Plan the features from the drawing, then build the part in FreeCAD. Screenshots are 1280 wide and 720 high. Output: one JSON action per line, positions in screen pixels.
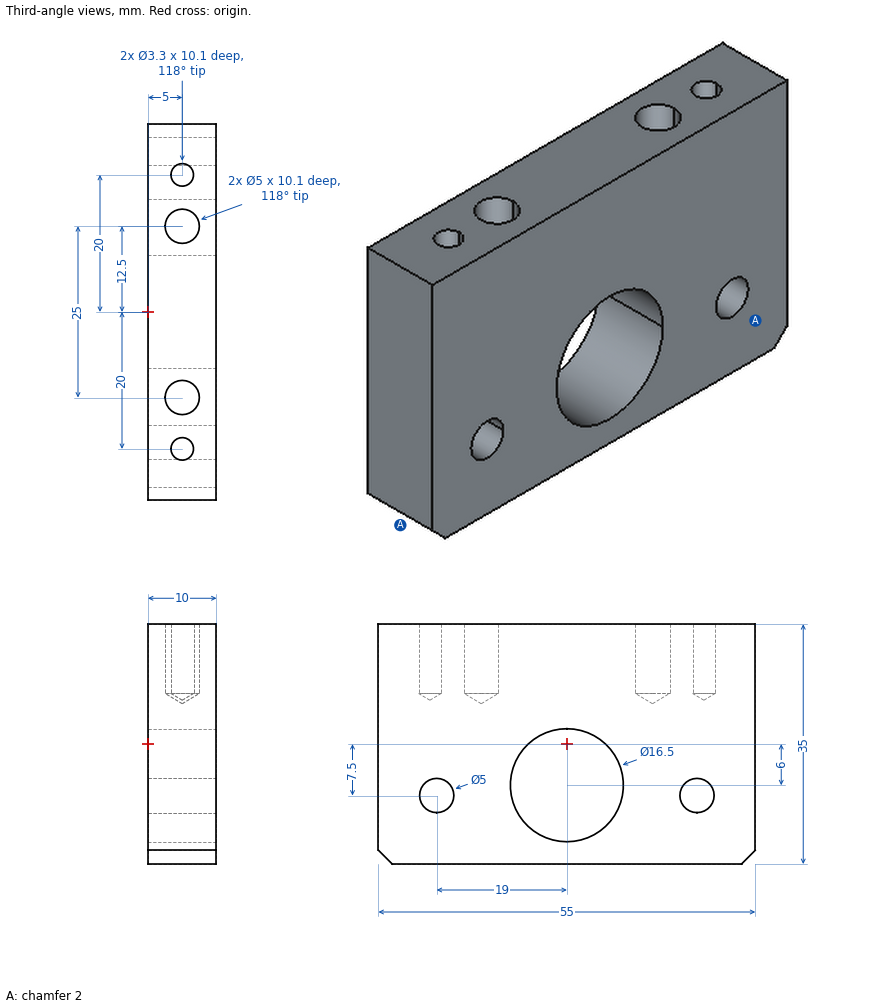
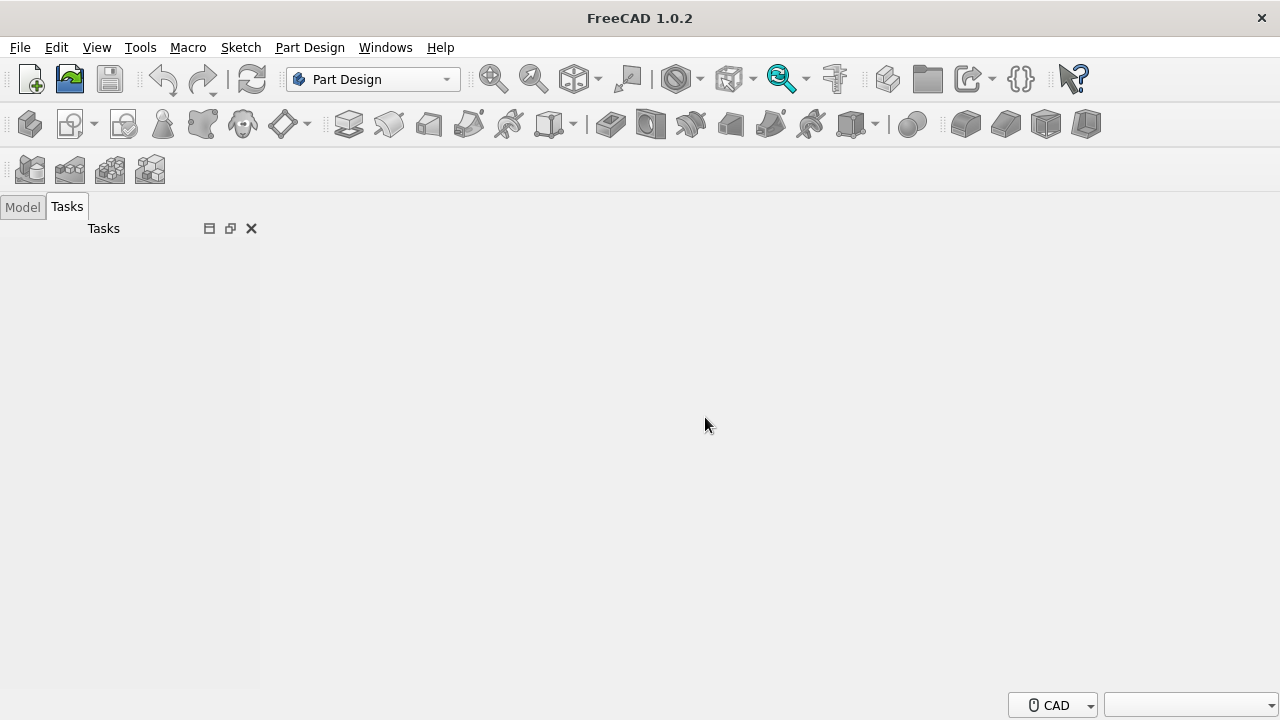
{"action": "left_click", "coordinate": [30, 80]}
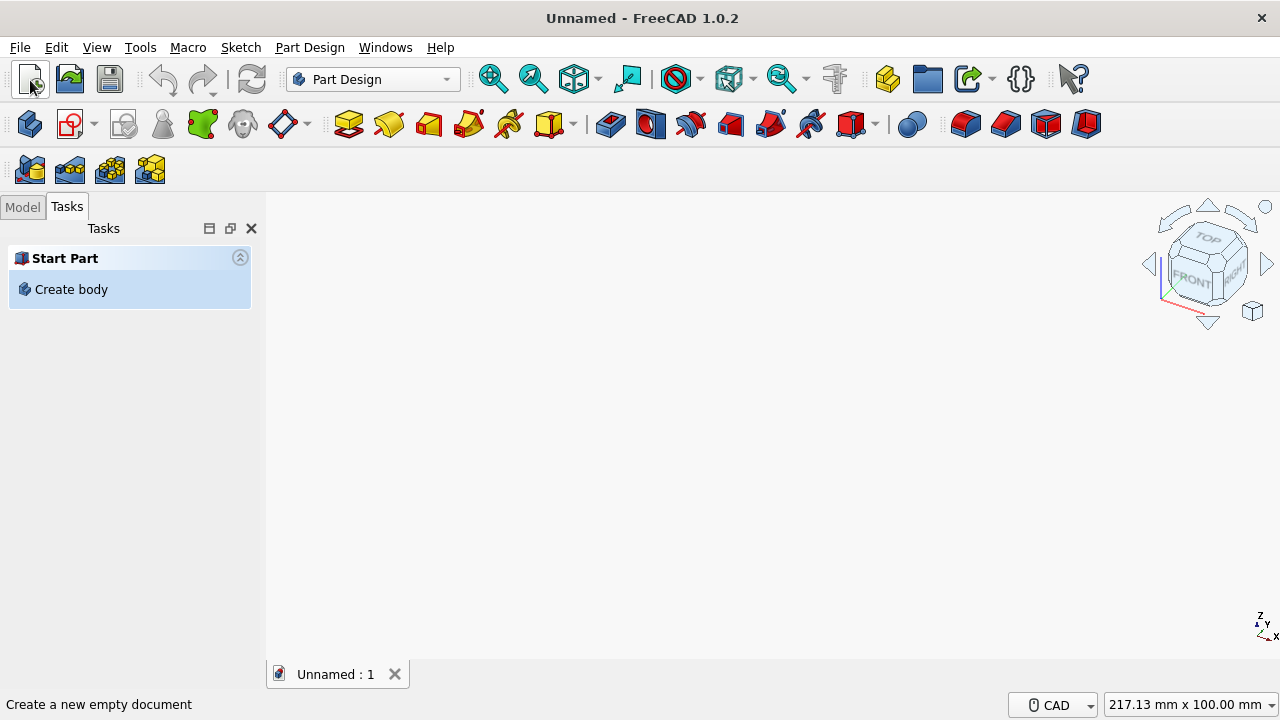
{"action": "left_click", "coordinate": [70, 124]}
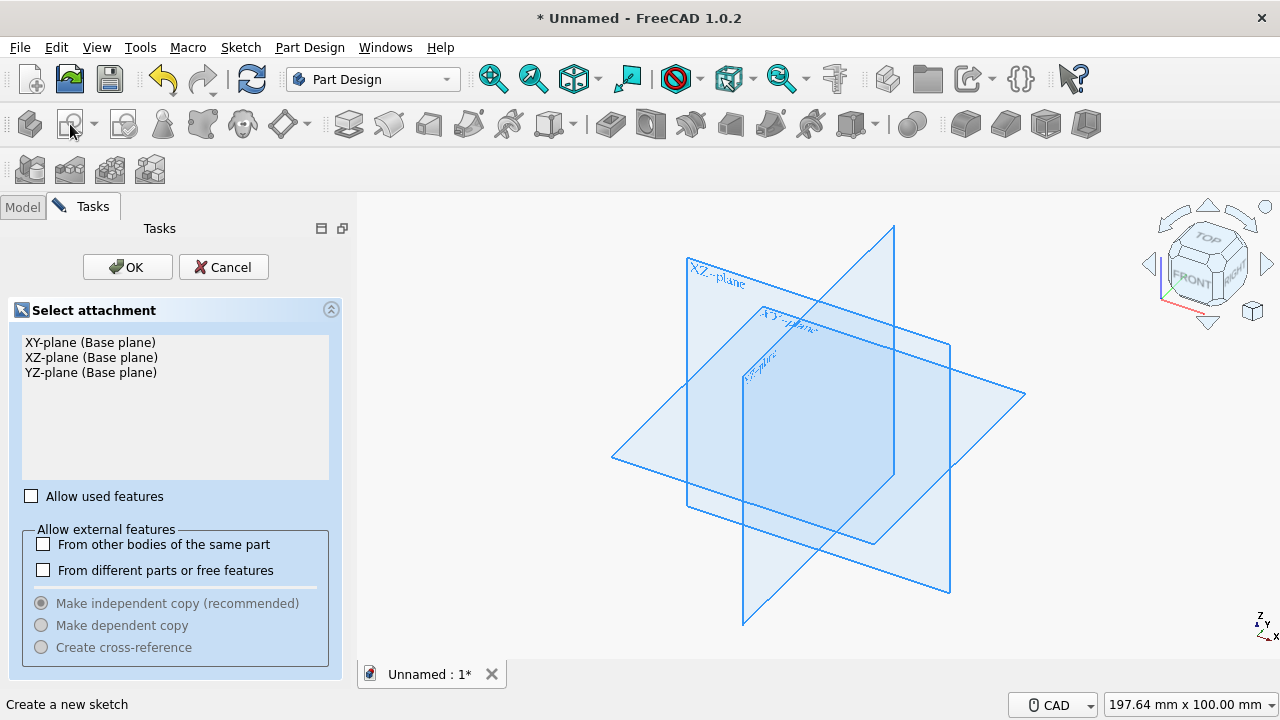
{"action": "left_click", "coordinate": [82, 372]}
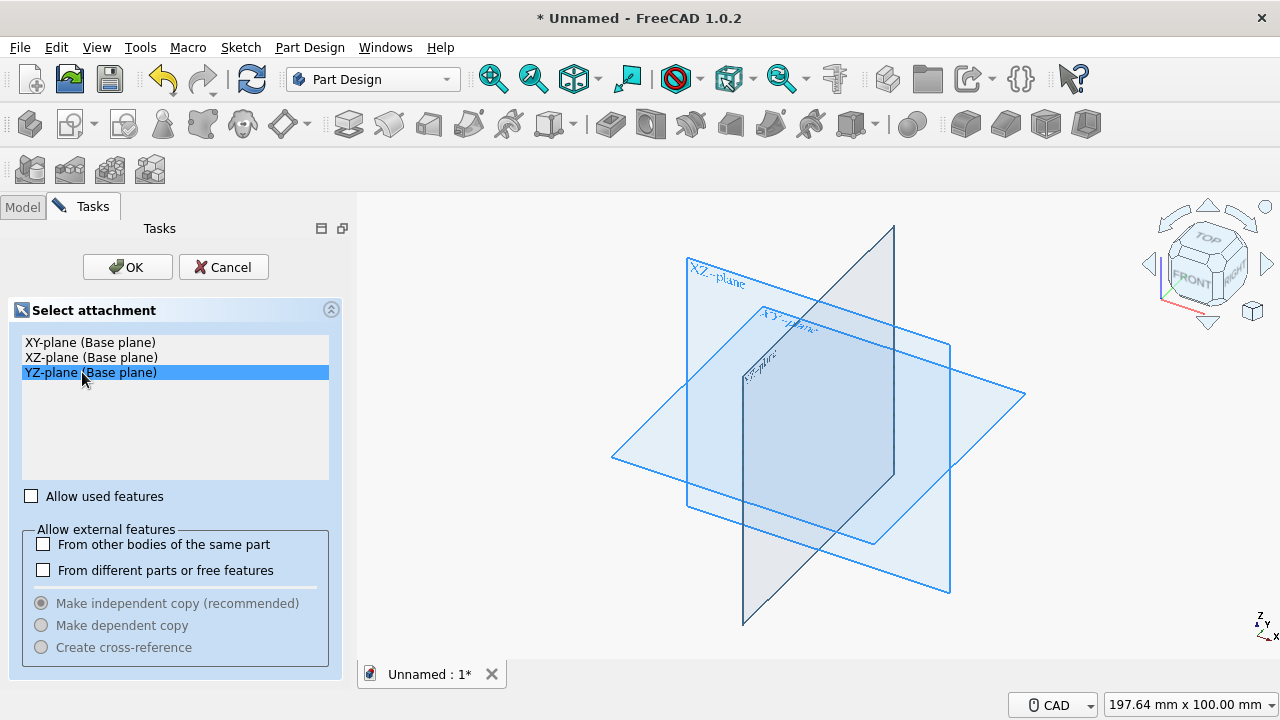
{"action": "left_click", "coordinate": [128, 267]}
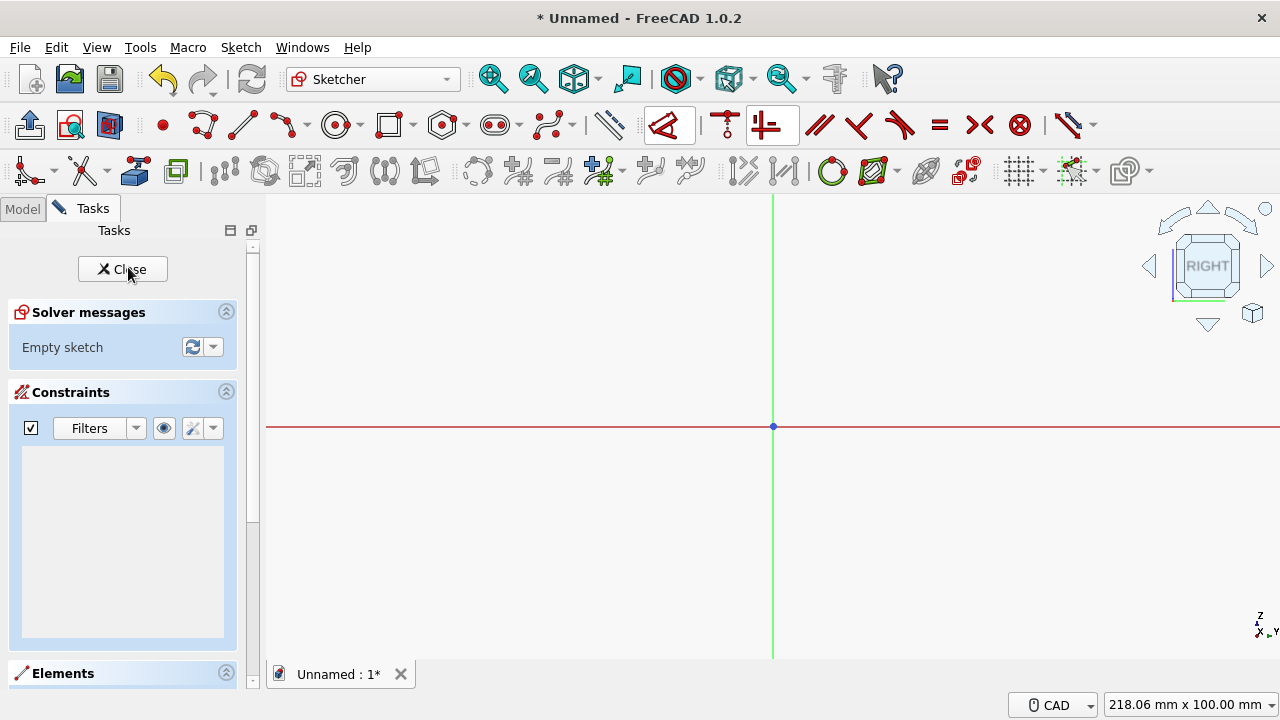
{"action": "scroll", "coordinate": [856, 426], "scroll_direction": "up", "scroll_amount": 3}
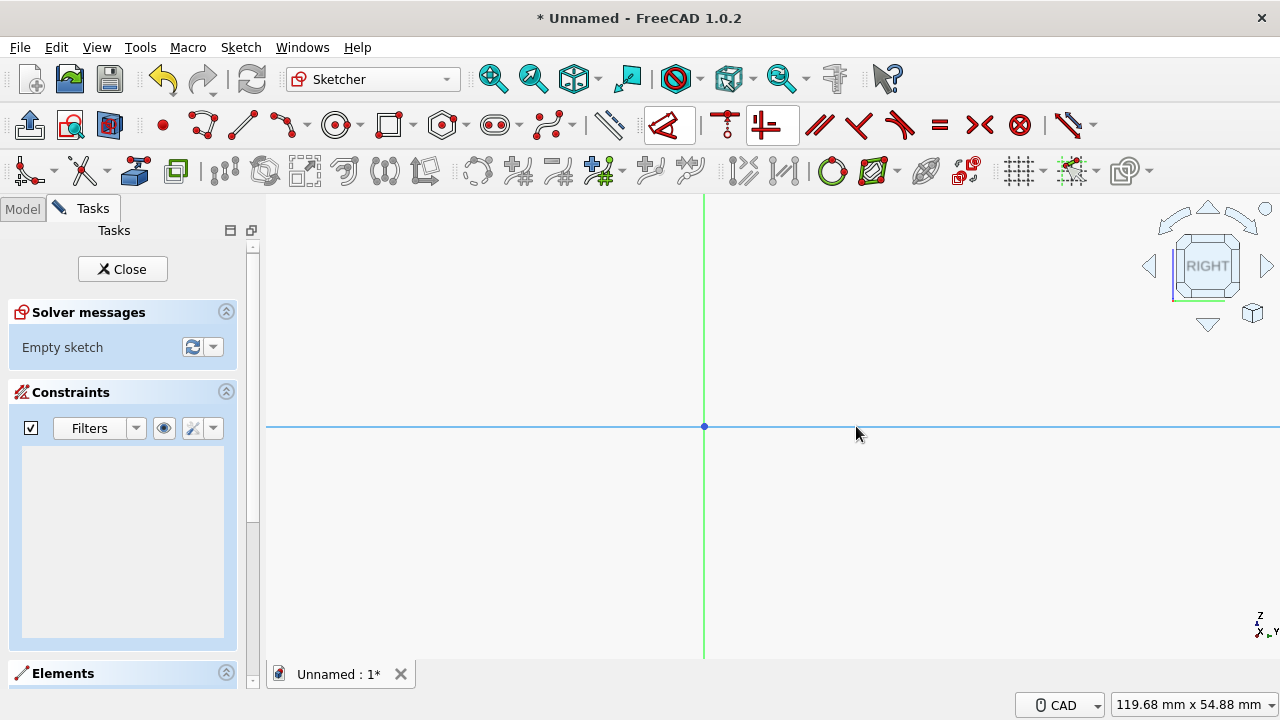
{"action": "key", "text": "g v"}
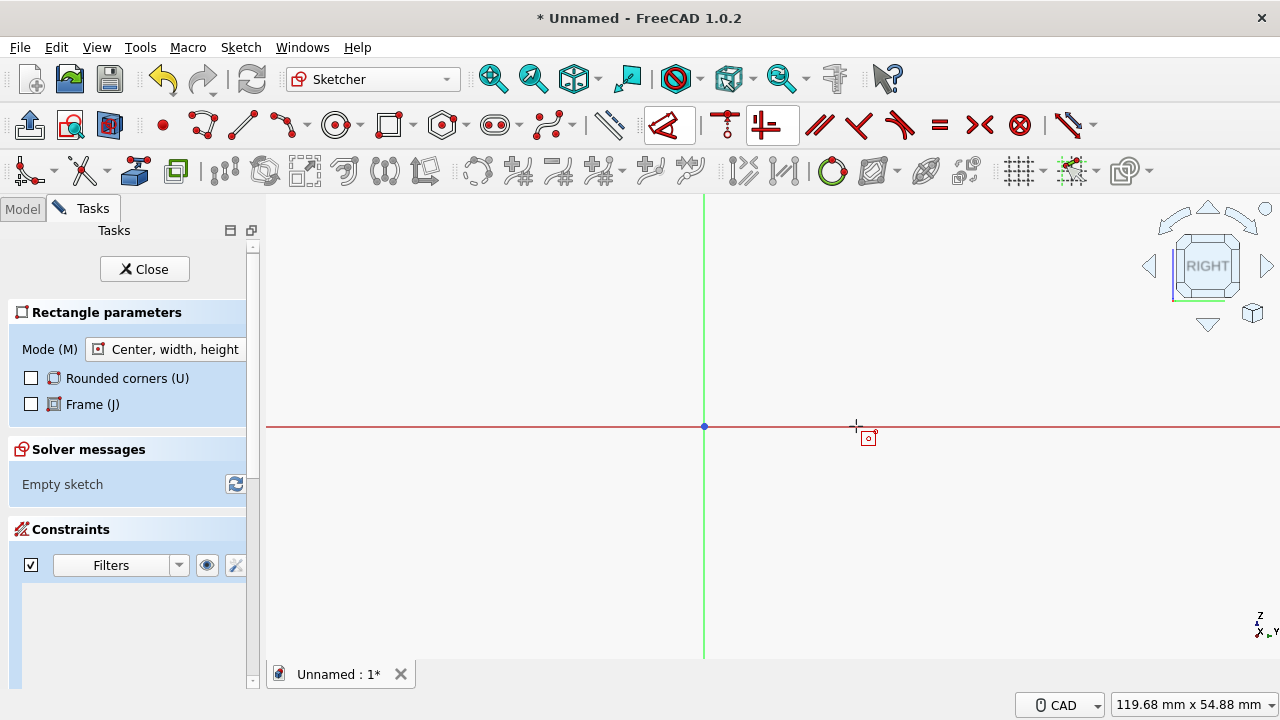
{"action": "left_click", "coordinate": [704, 426]}
{"action": "mouse_move", "coordinate": [937, 278]}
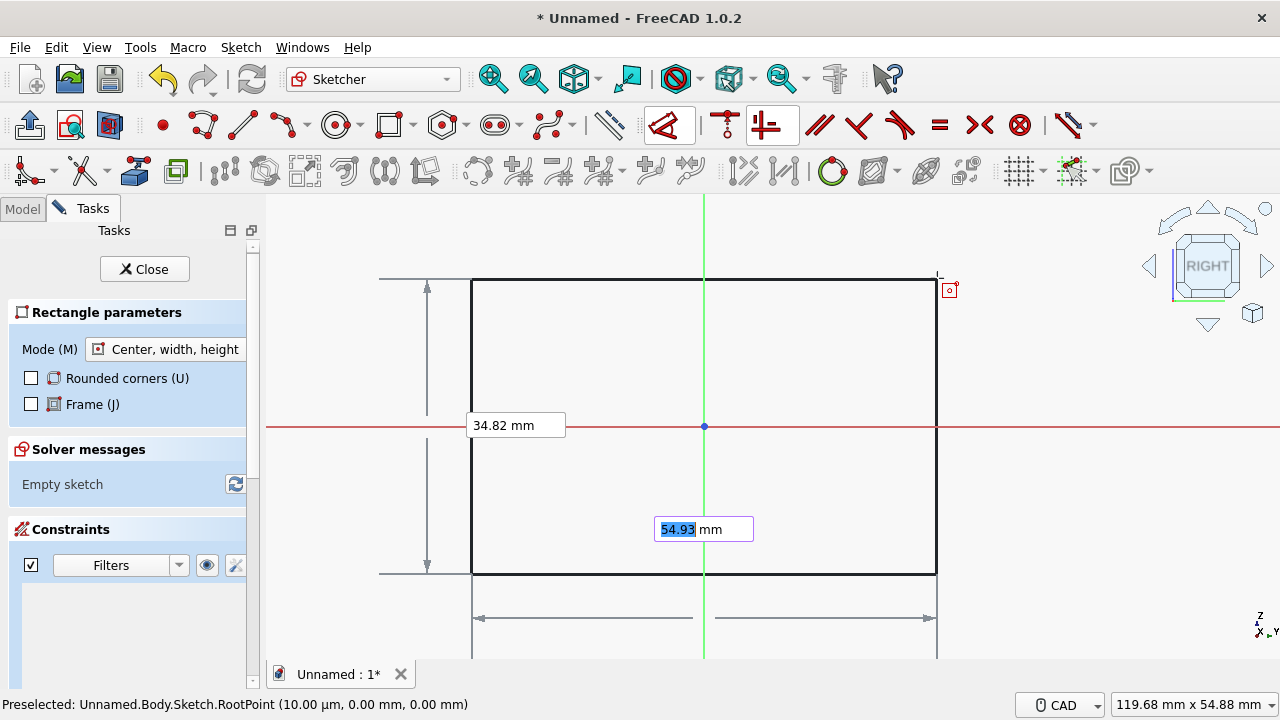
{"action": "type", "text": "55"}
{"action": "key", "text": "Tab"}
{"action": "type", "text": "35"}
{"action": "key", "text": "Return"}
{"action": "key", "text": "Escape"}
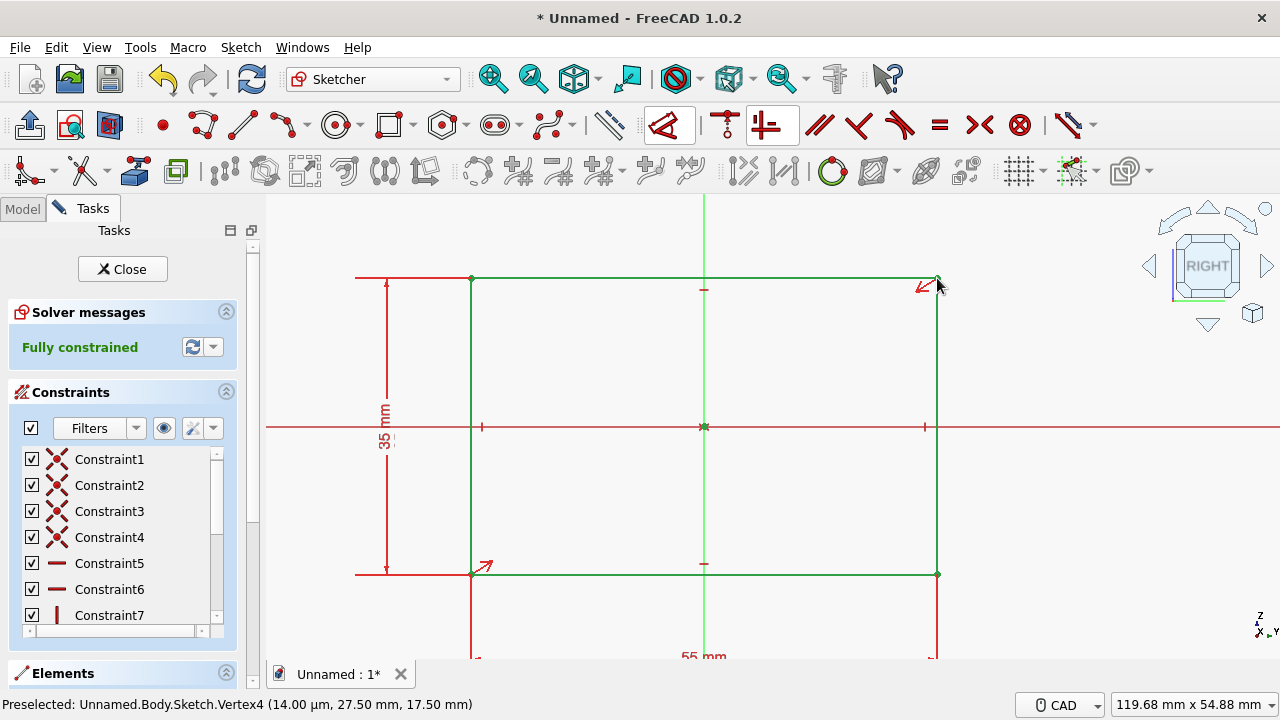
{"action": "left_click", "coordinate": [123, 269]}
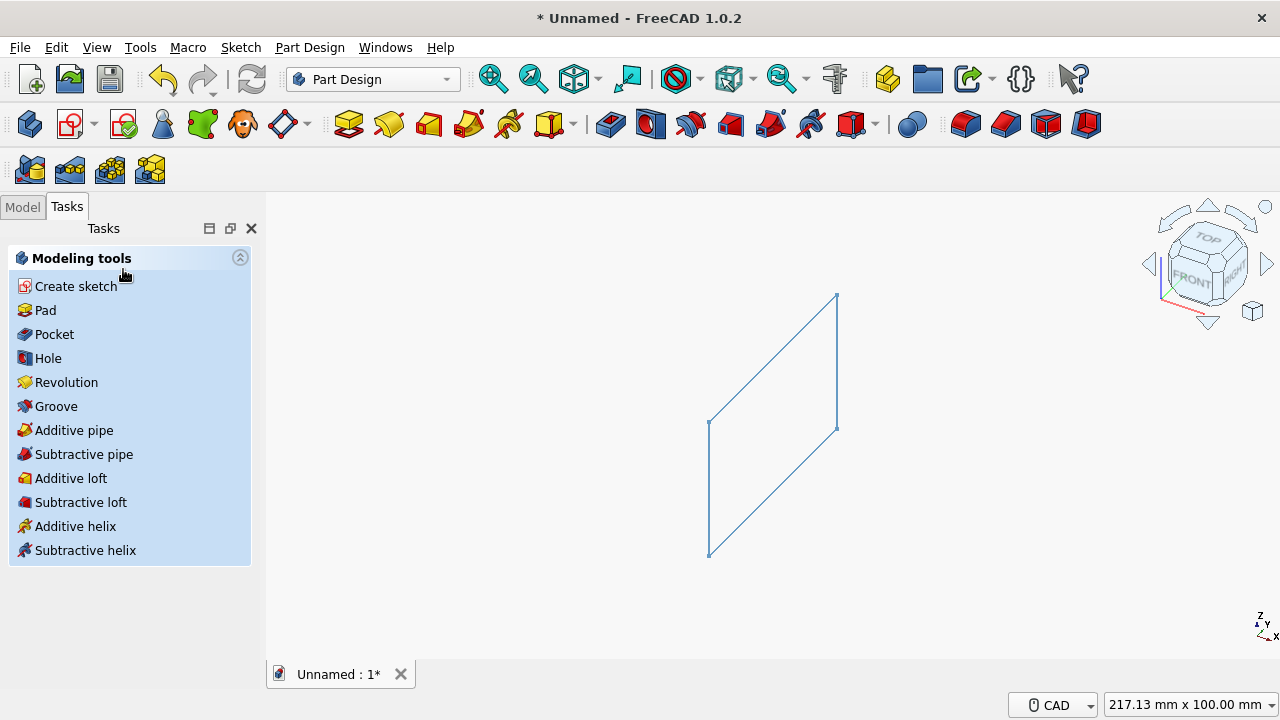
{"action": "left_click", "coordinate": [350, 124]}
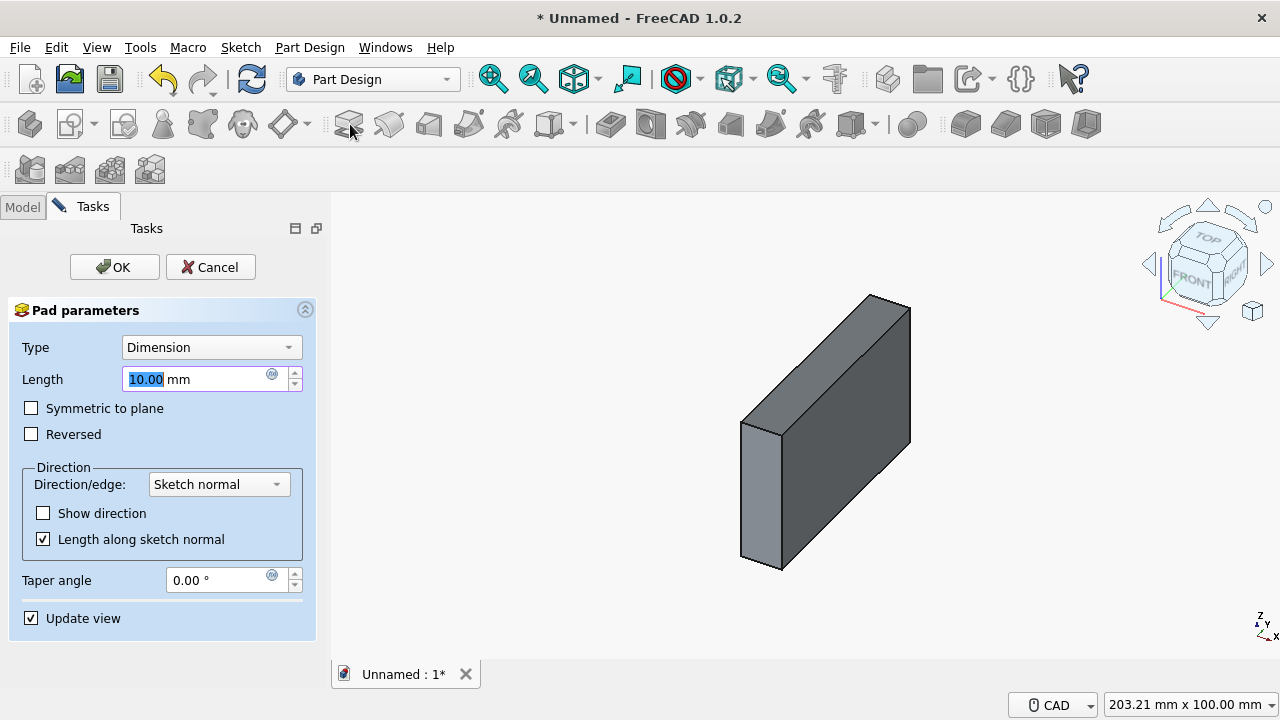
{"action": "type", "text": "10"}
{"action": "key", "text": "Tab"}